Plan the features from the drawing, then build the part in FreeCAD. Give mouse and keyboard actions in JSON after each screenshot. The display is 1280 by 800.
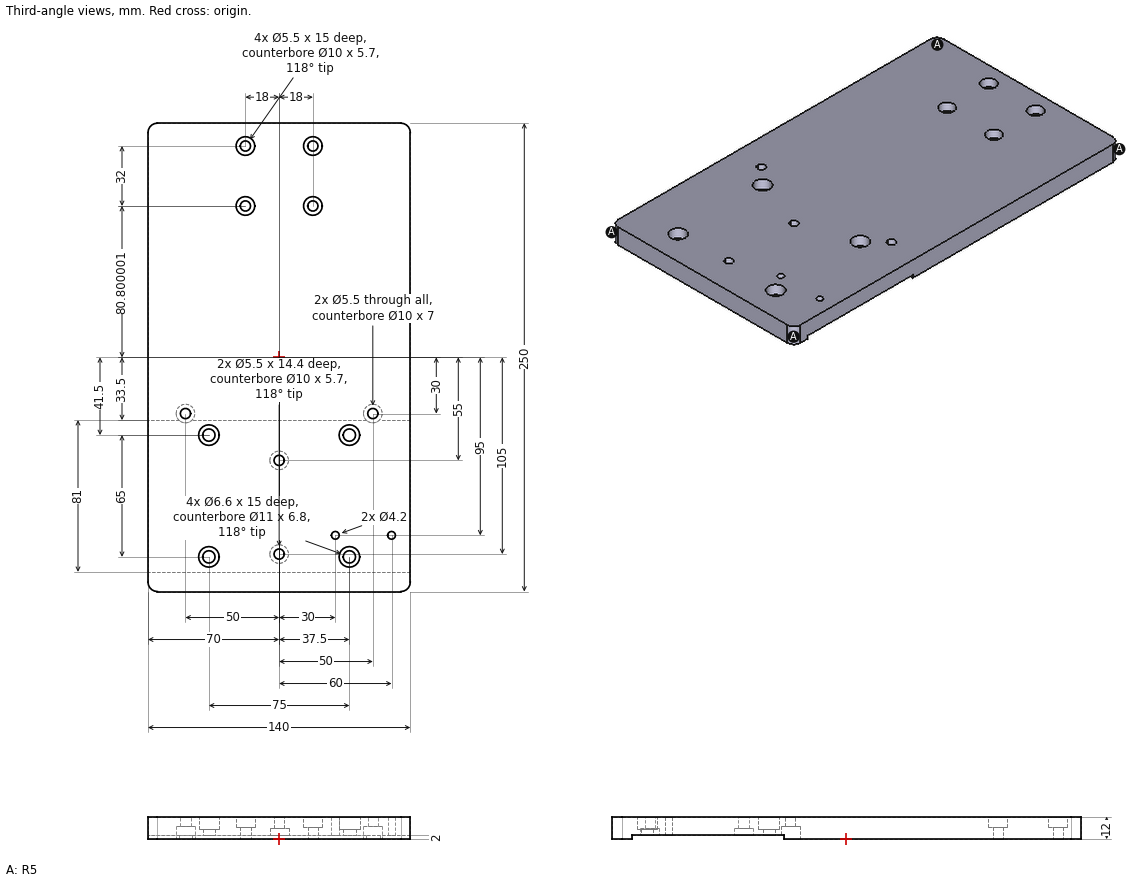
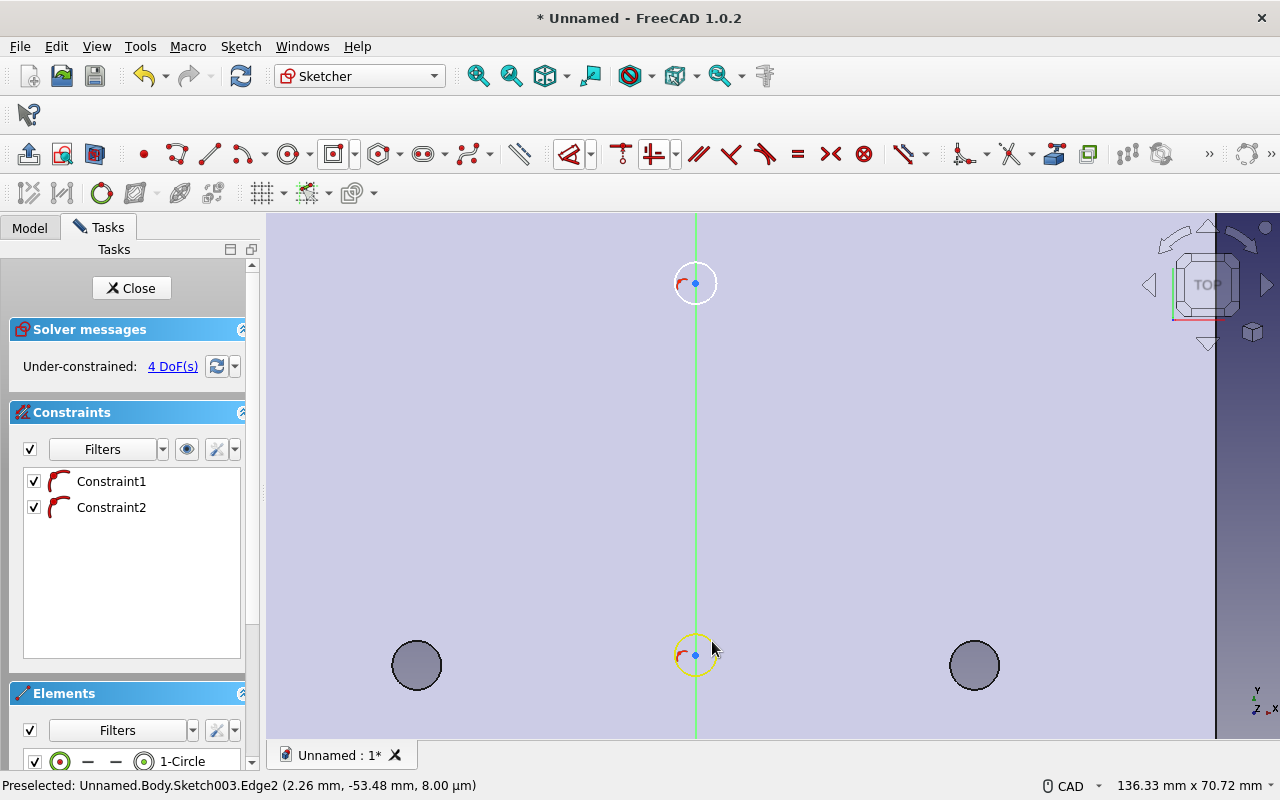
{"action": "left_click", "coordinate": [710, 640]}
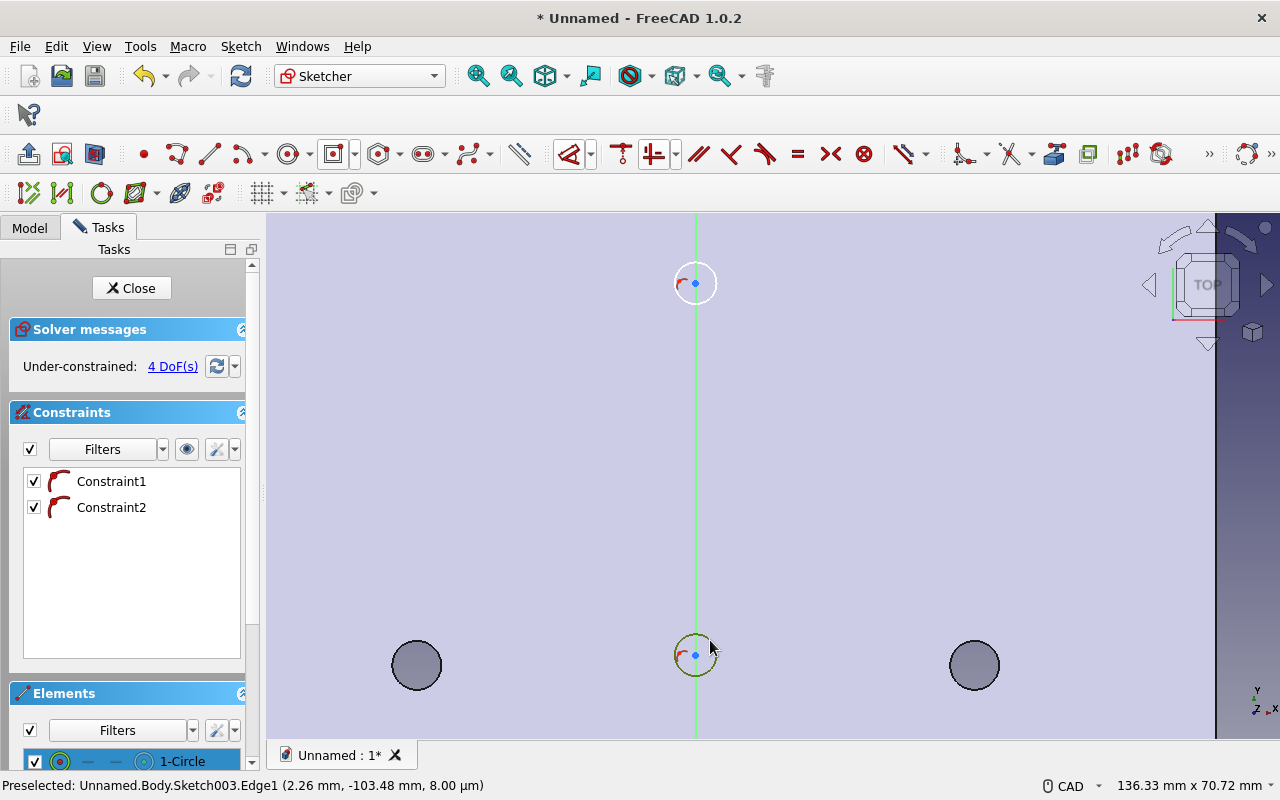
{"action": "left_click", "coordinate": [710, 268]}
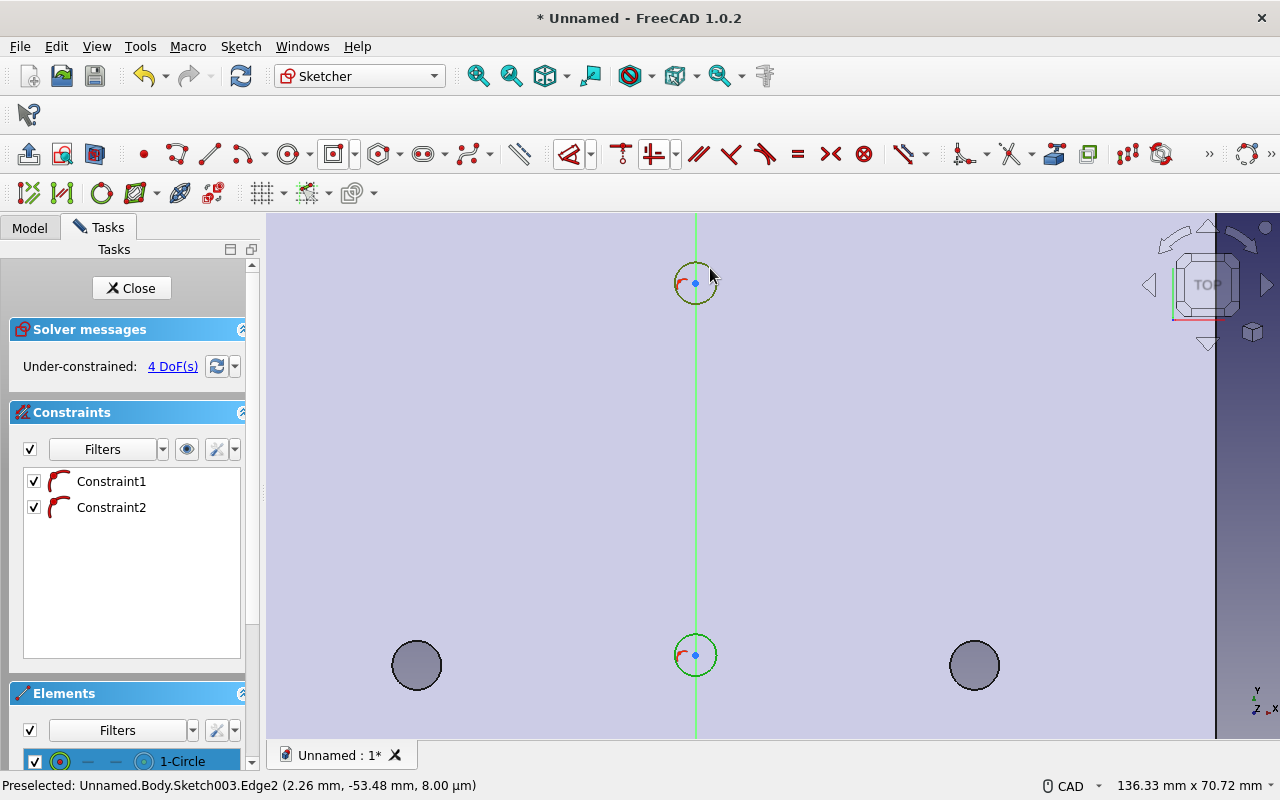
{"action": "left_click", "coordinate": [798, 154]}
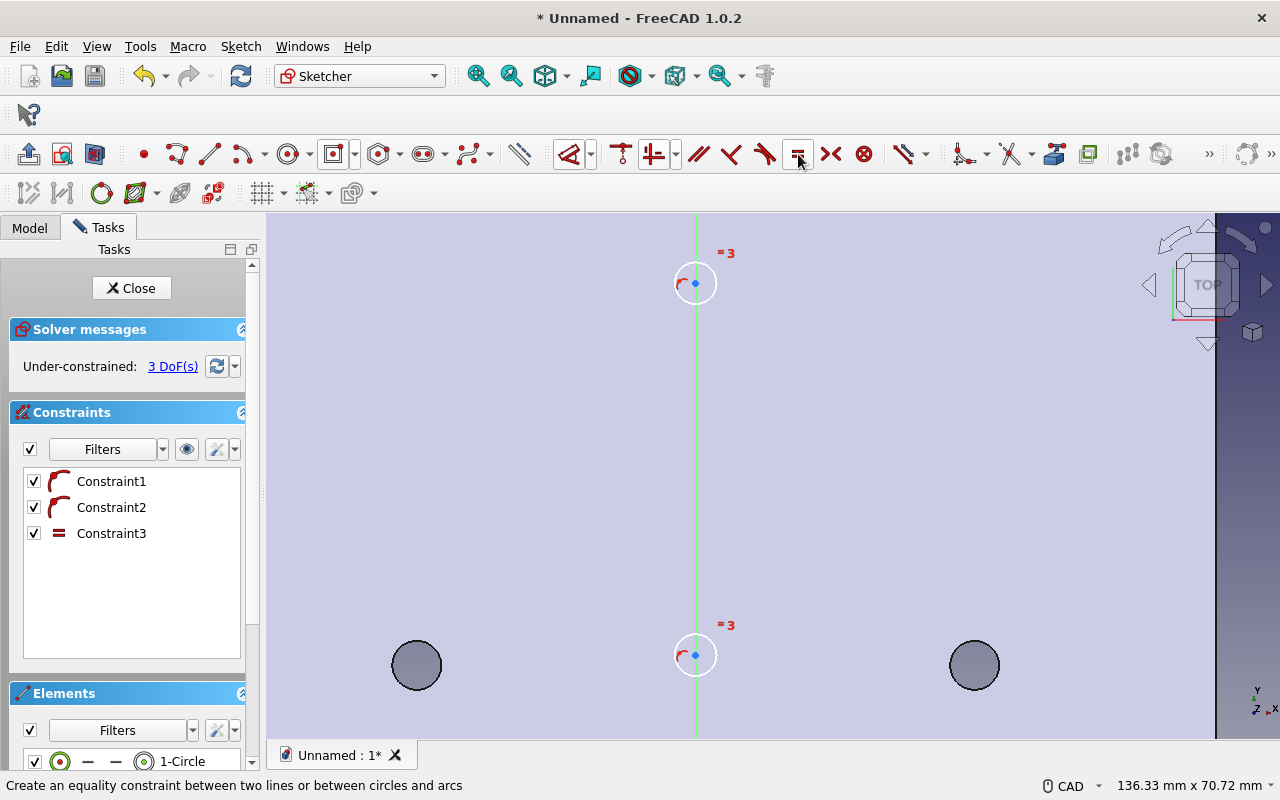
{"action": "left_click", "coordinate": [710, 640]}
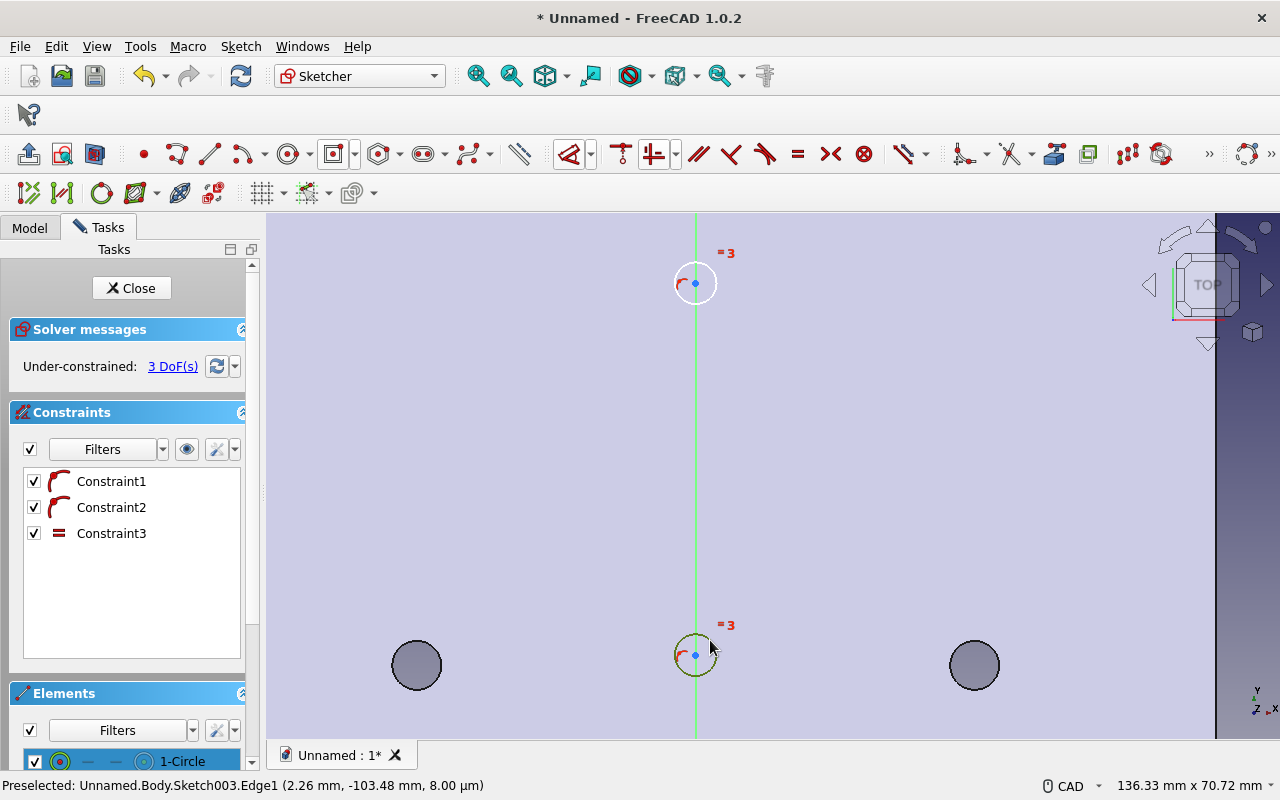
{"action": "key", "text": "k o"}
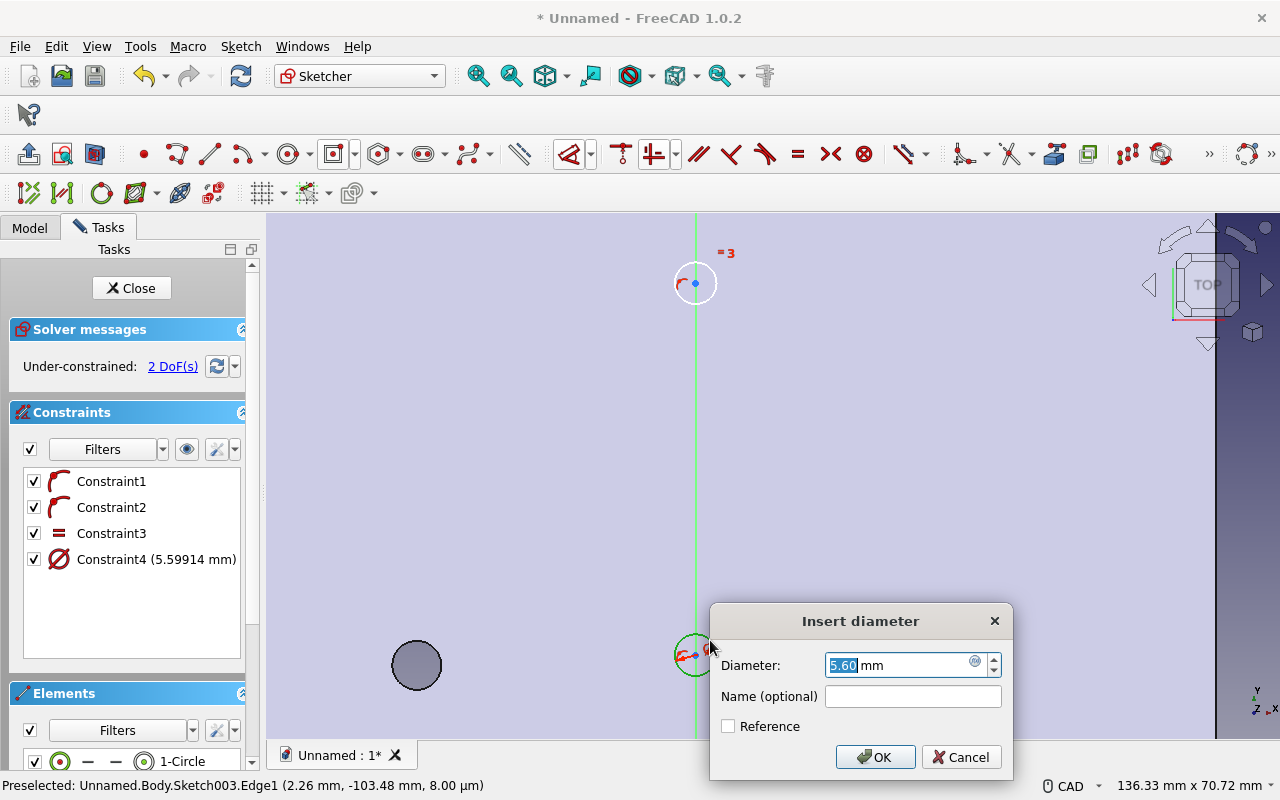
{"action": "type", "text": "5.5"}
{"action": "key", "text": "Return"}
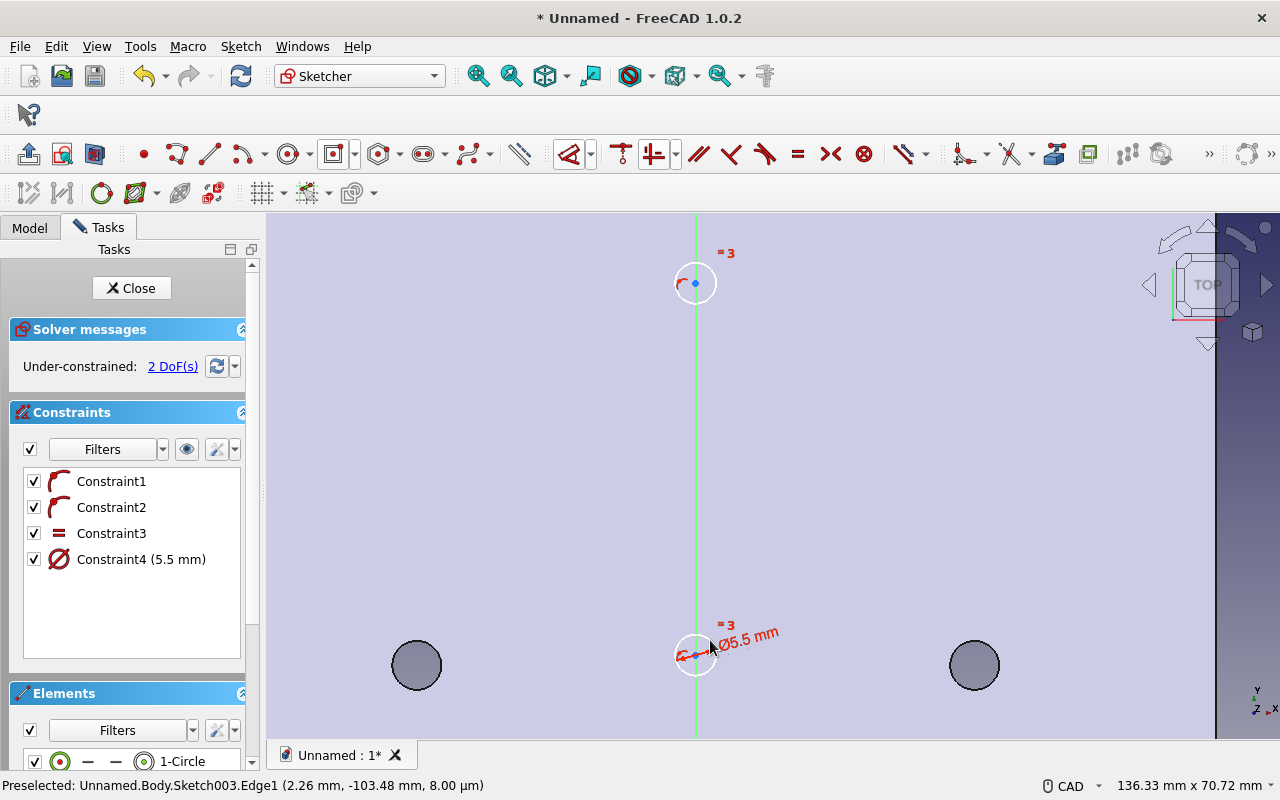
{"action": "left_click", "coordinate": [696, 283]}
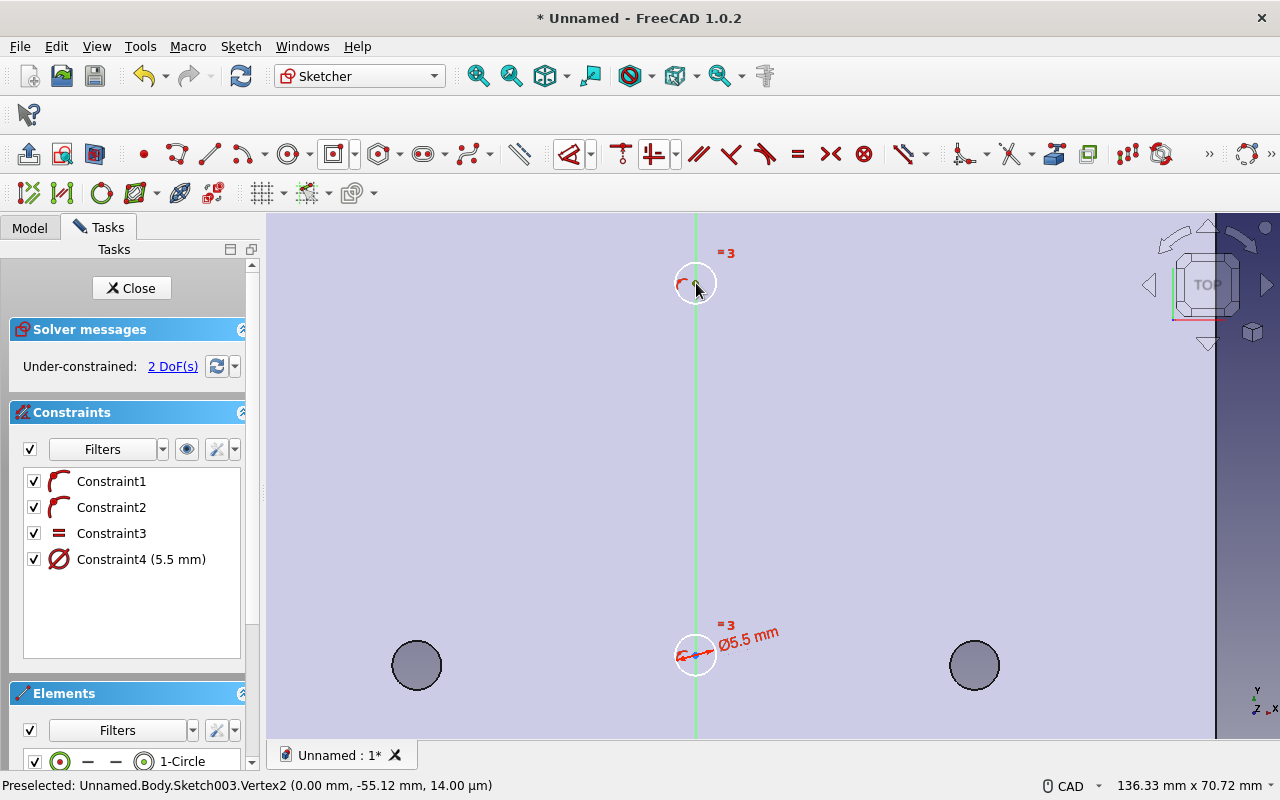
{"action": "left_click", "coordinate": [590, 154]}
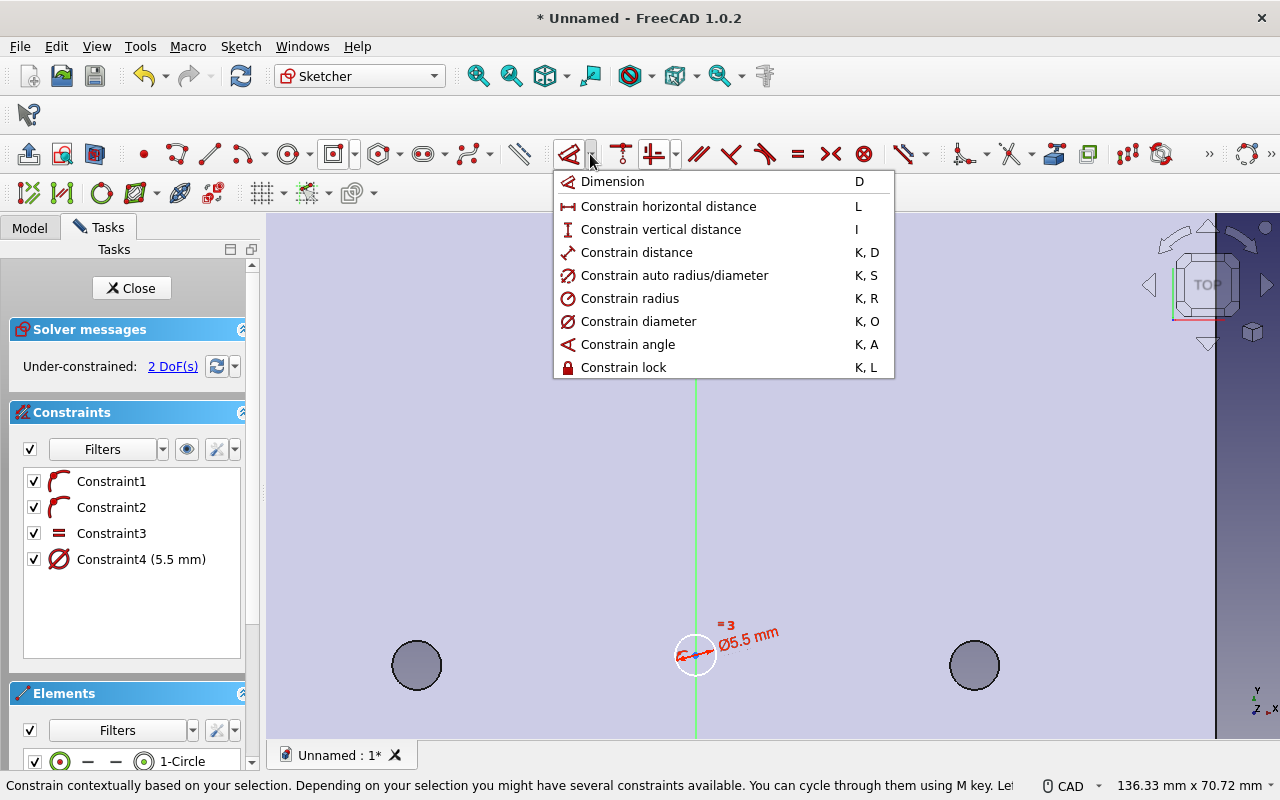
{"action": "left_click", "coordinate": [724, 230]}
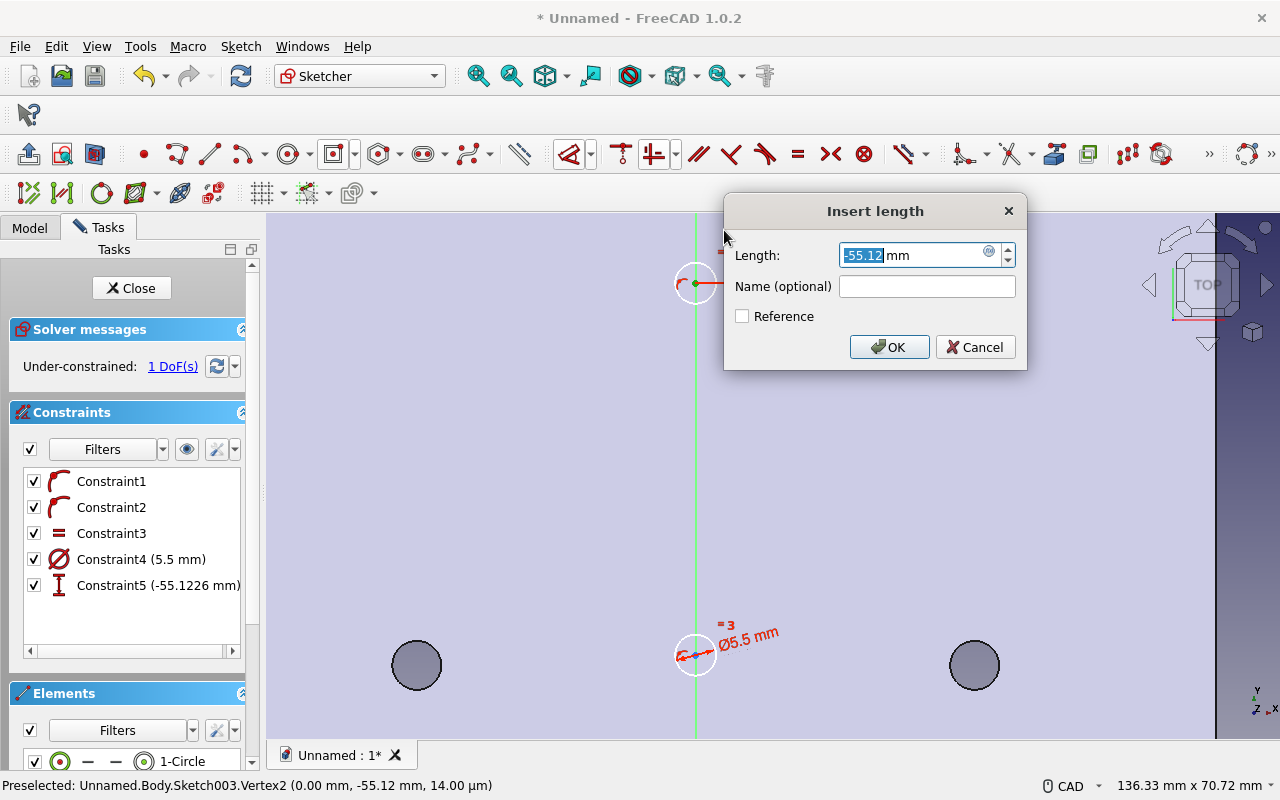
{"action": "type", "text": "-55"}
{"action": "key", "text": "Return"}